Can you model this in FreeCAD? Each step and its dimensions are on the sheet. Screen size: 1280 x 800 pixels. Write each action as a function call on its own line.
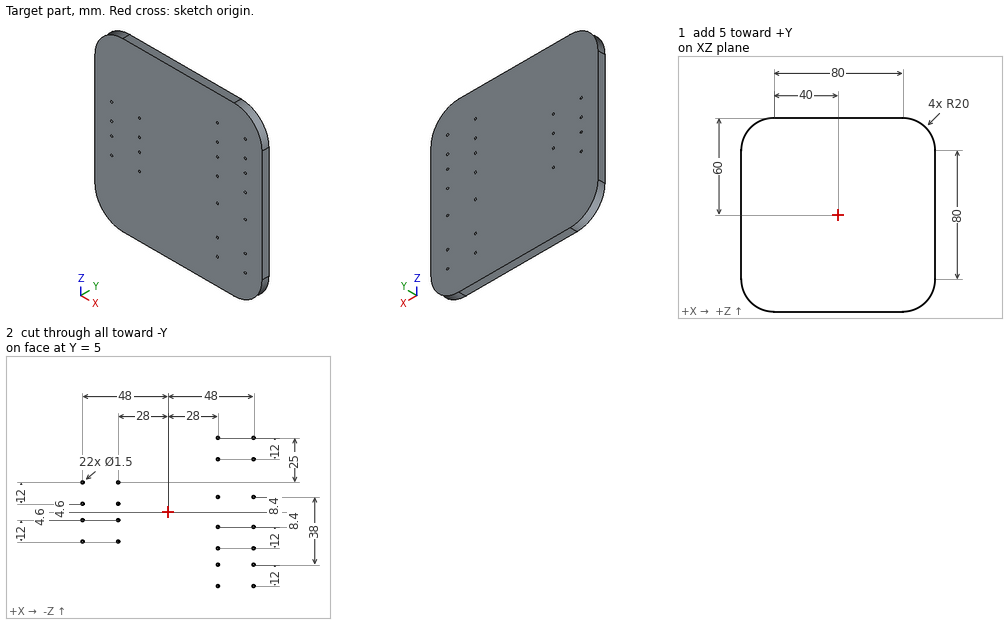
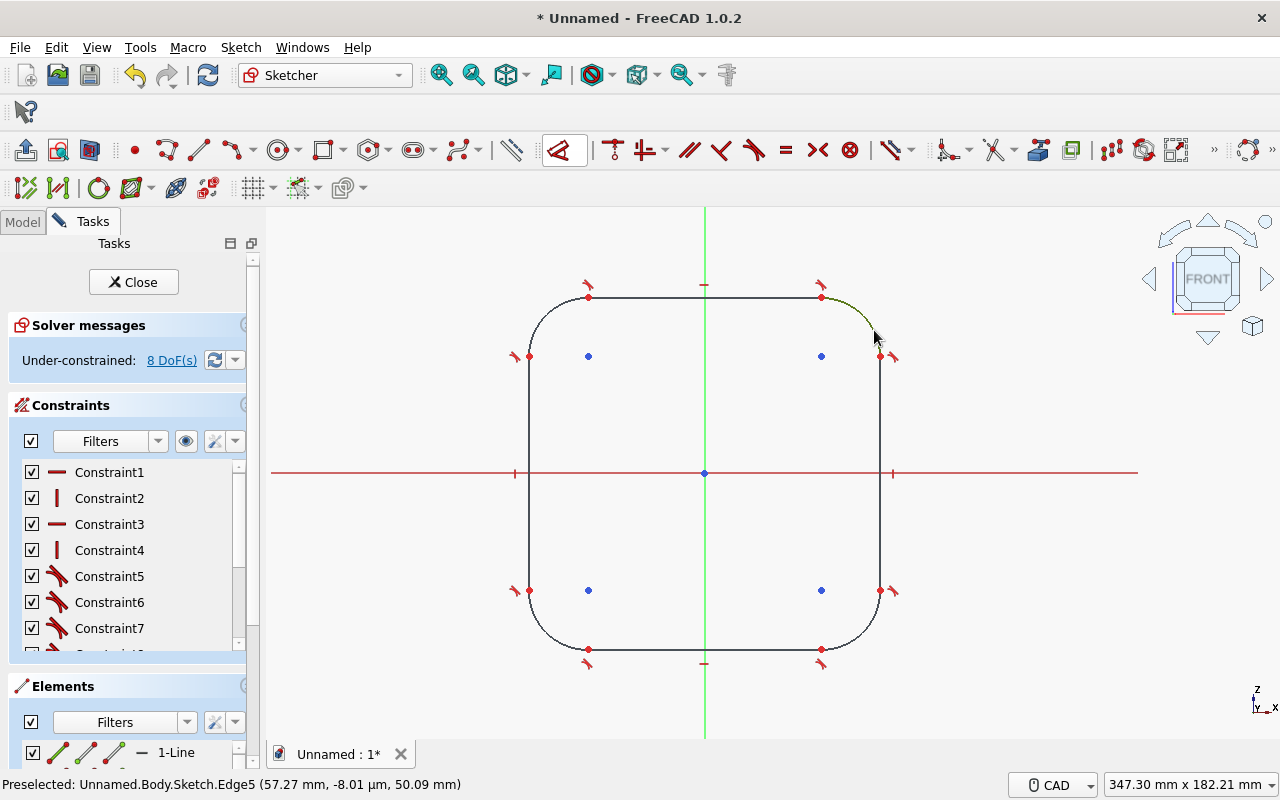
click(848, 644)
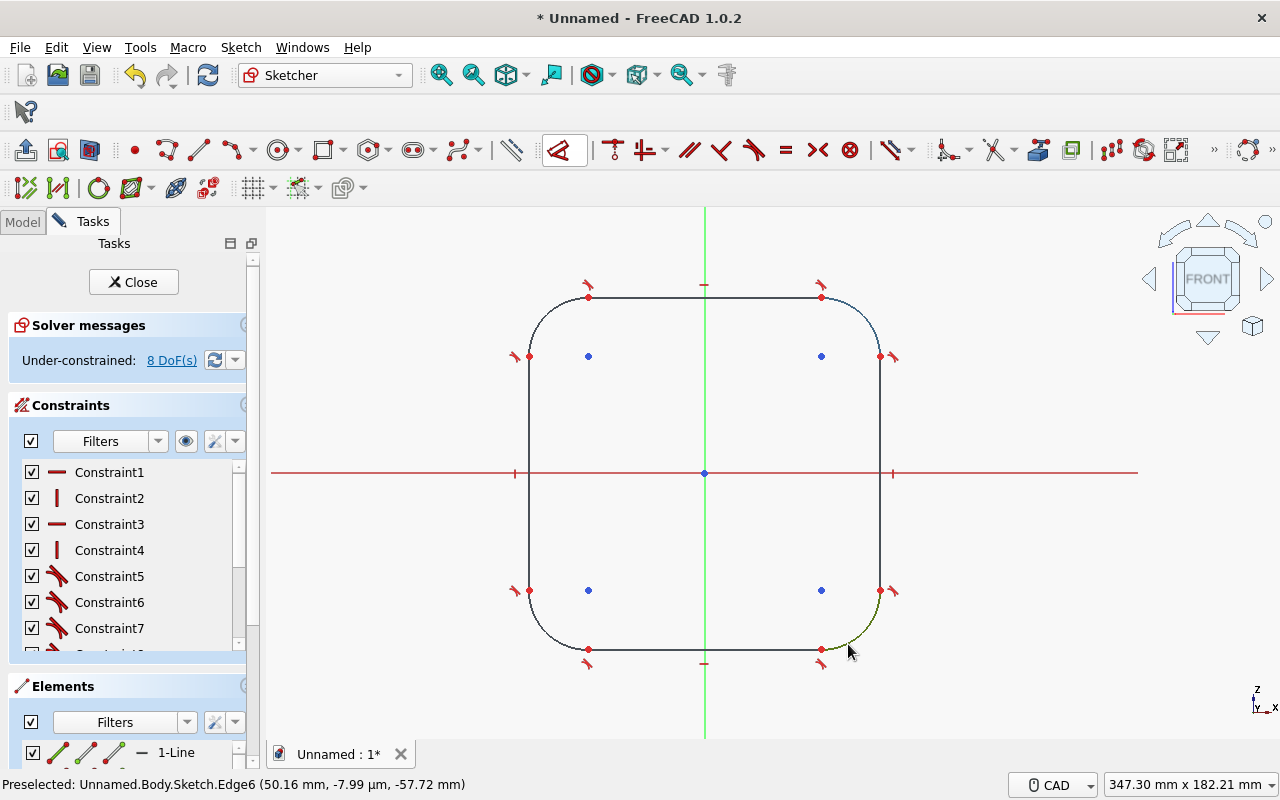
click(535, 618)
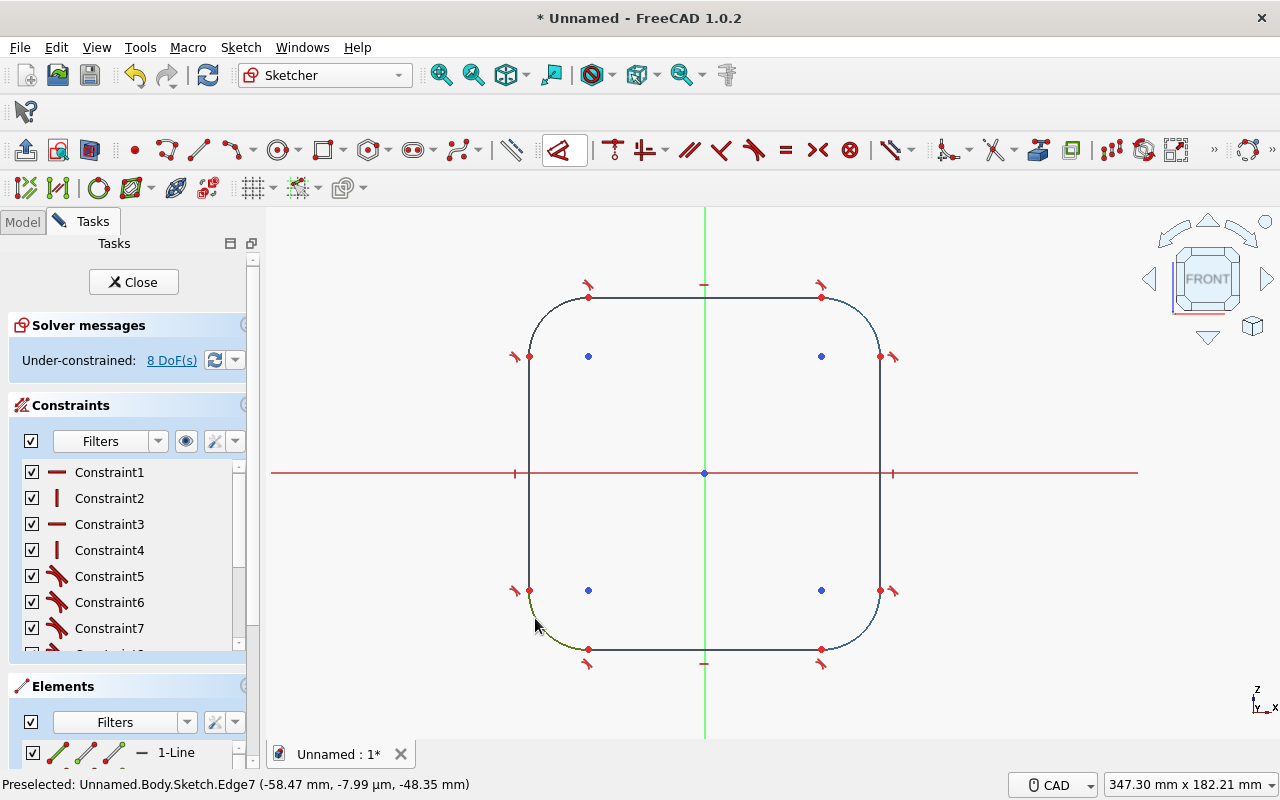
click(561, 304)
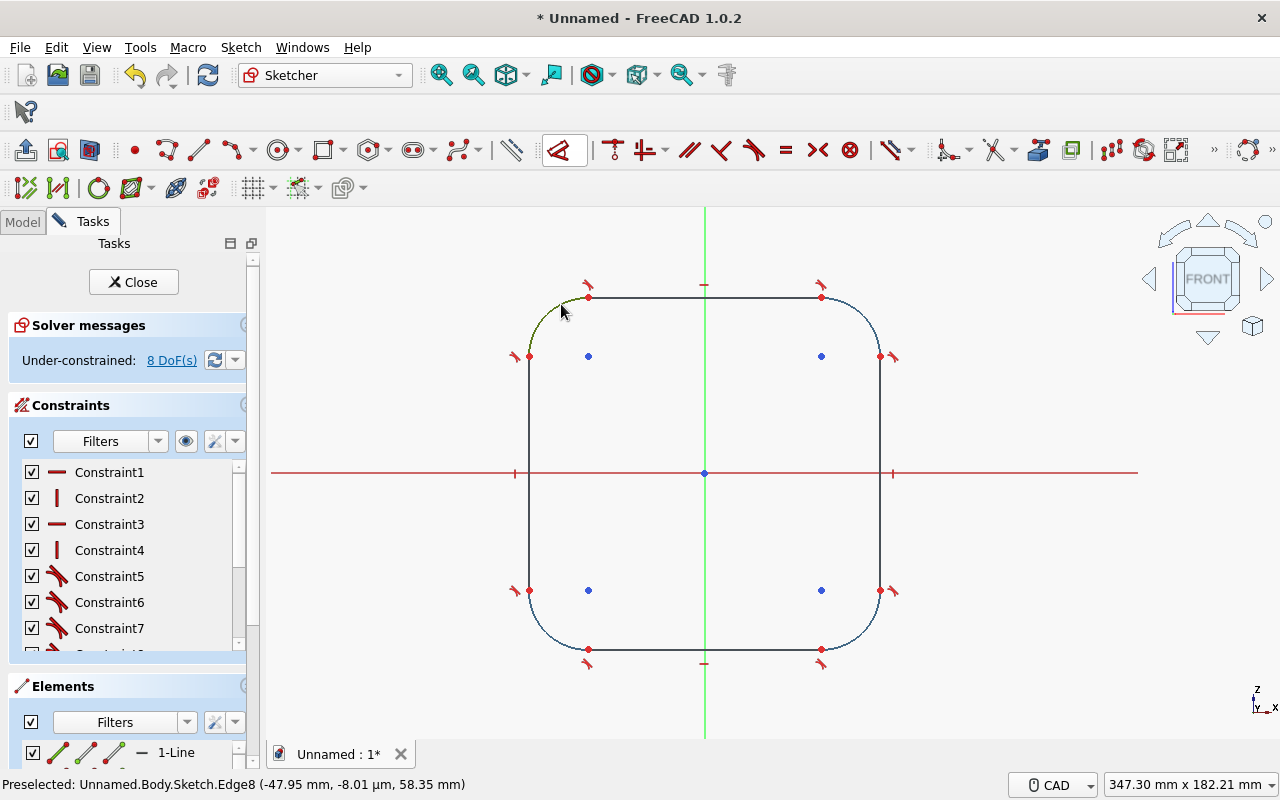
click(786, 150)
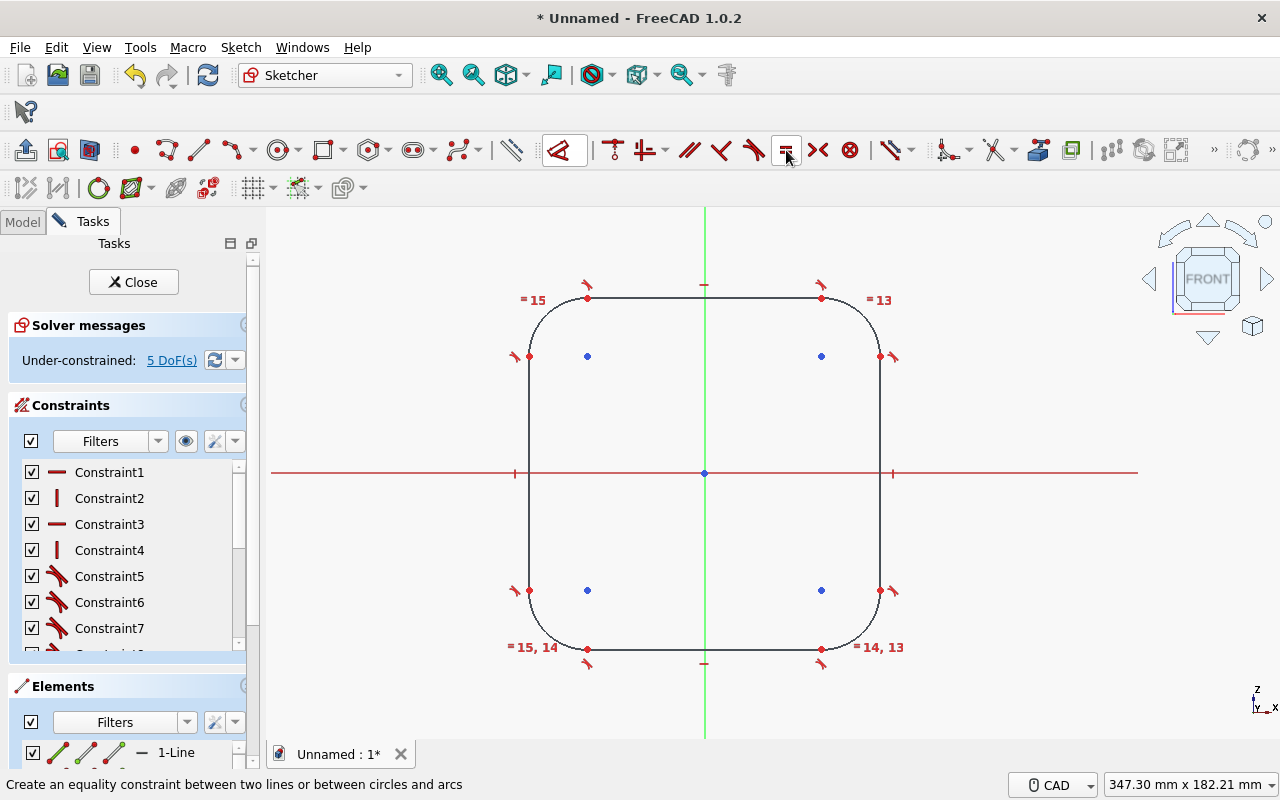
click(558, 150)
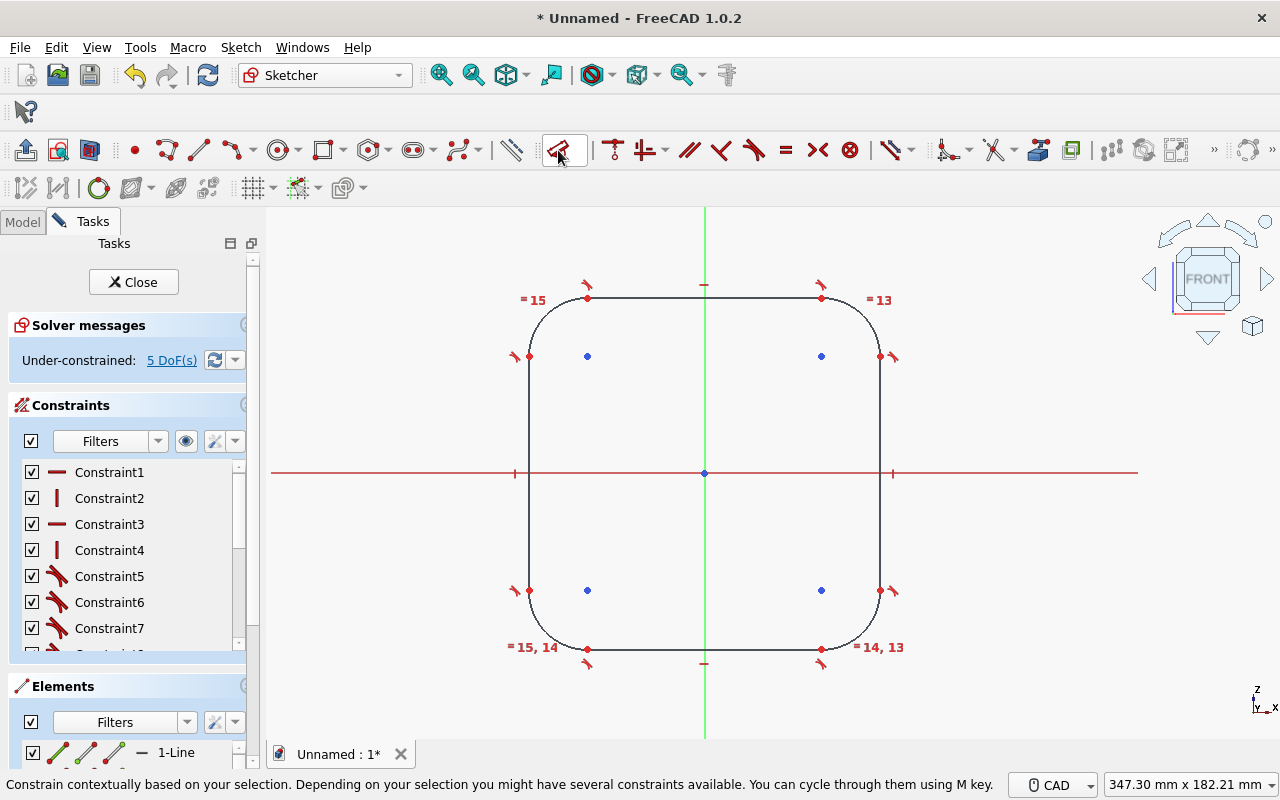
click(874, 330)
click(903, 315)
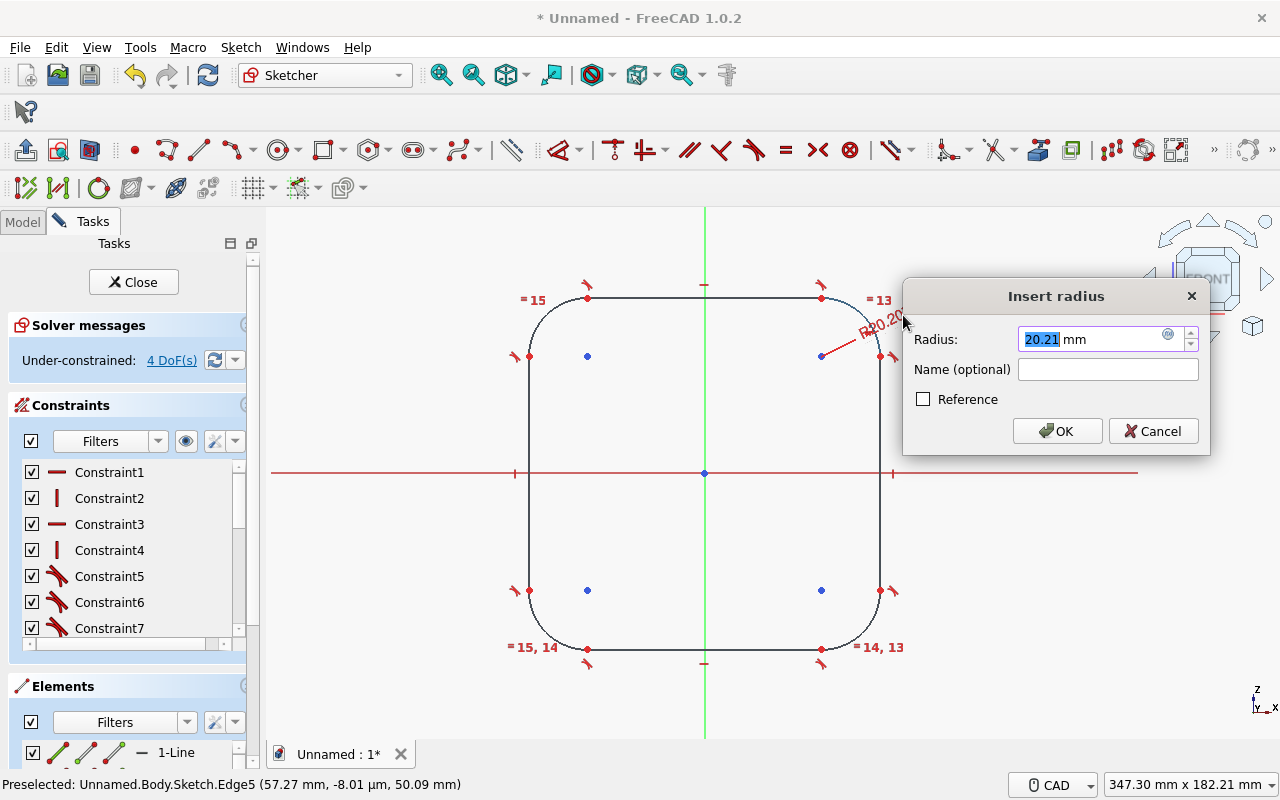
text(20)
key(Return)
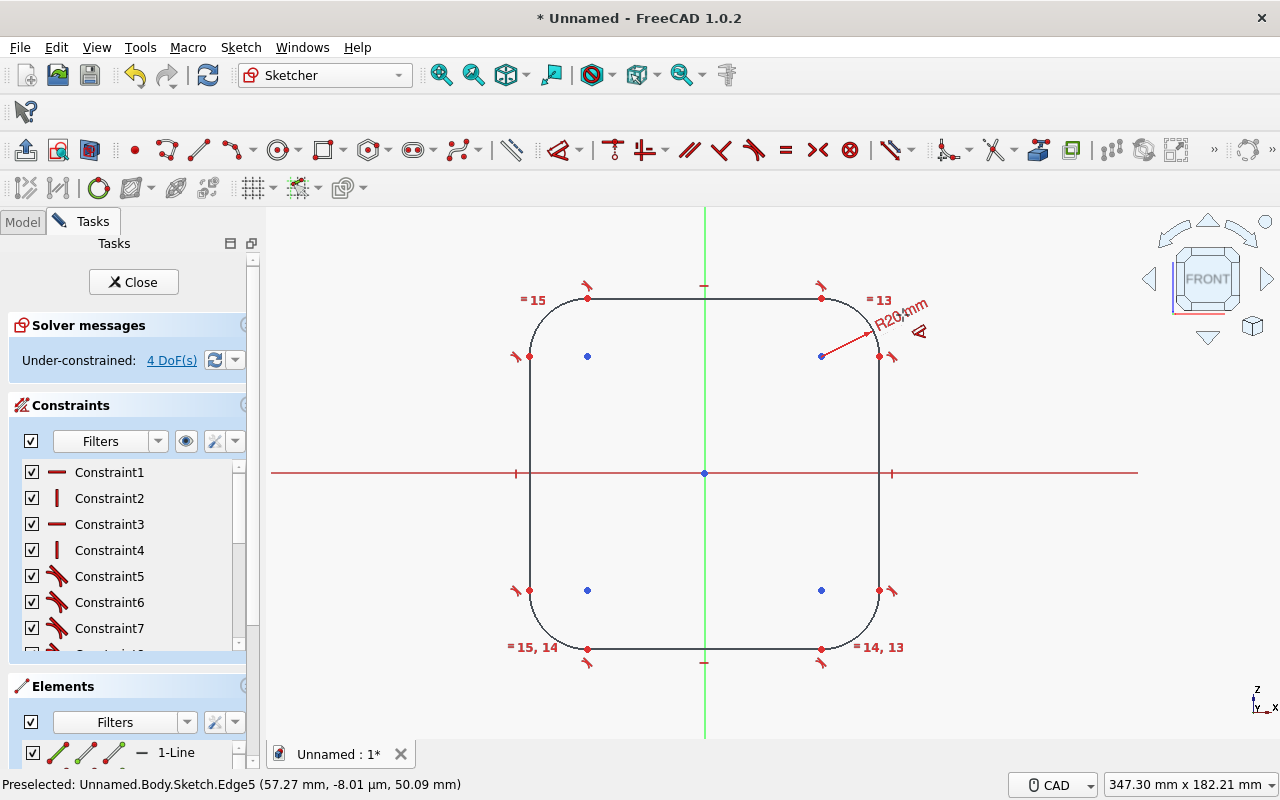
click(658, 299)
click(651, 265)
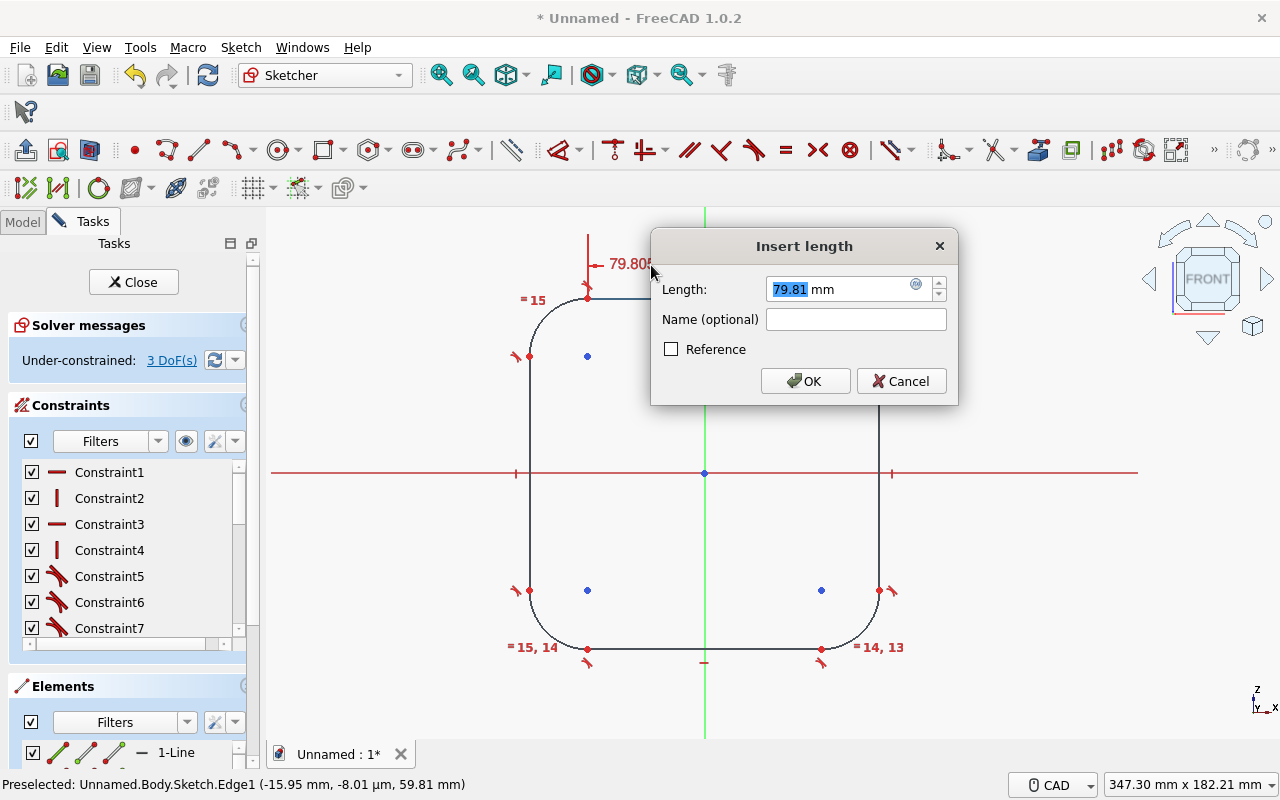
text(80)
key(Return)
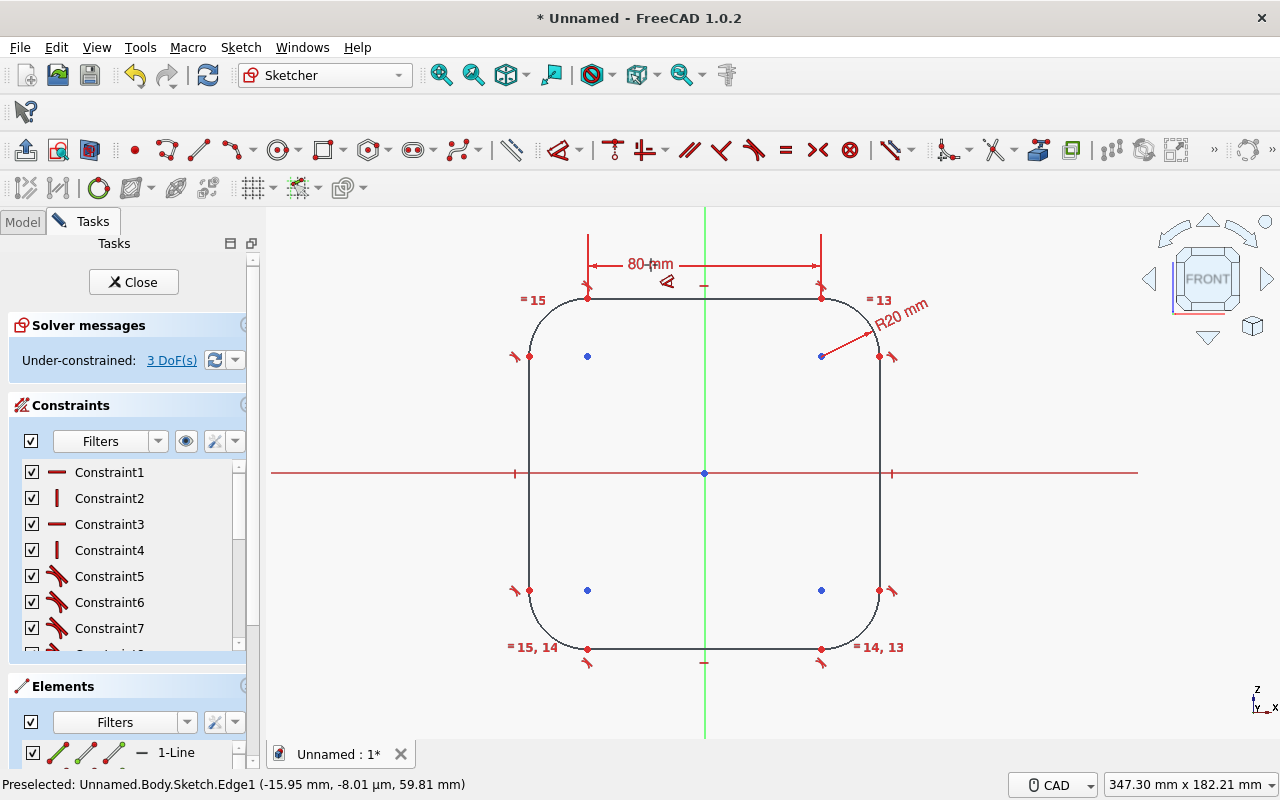
click(880, 427)
click(914, 420)